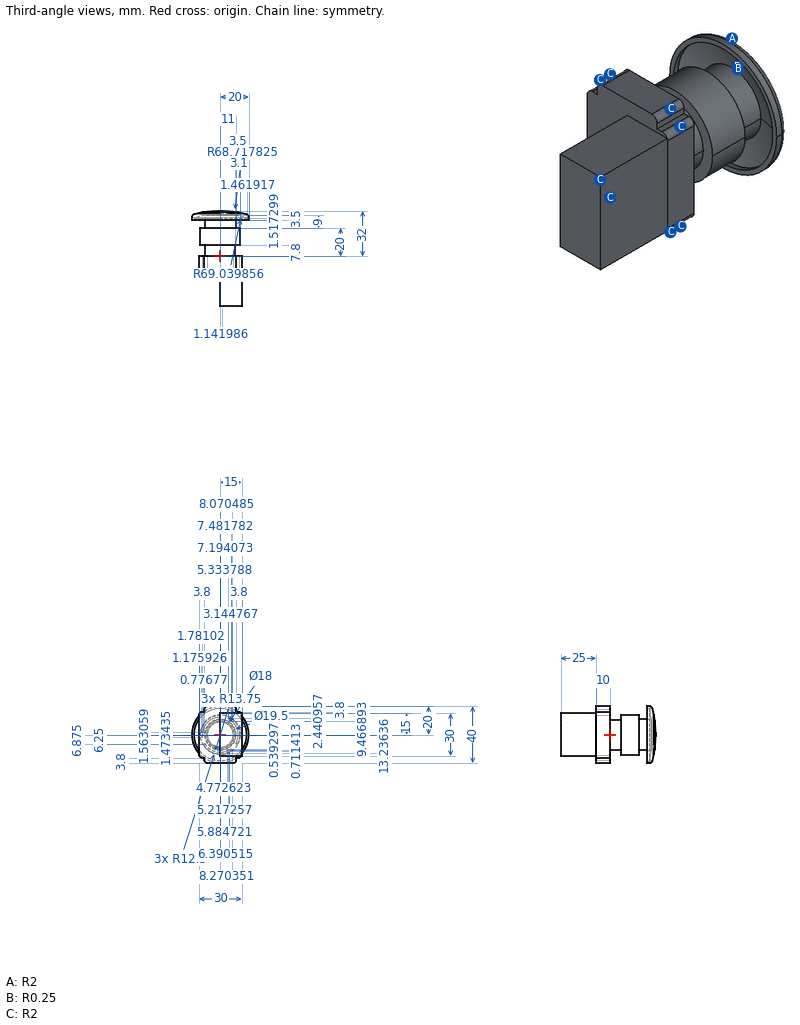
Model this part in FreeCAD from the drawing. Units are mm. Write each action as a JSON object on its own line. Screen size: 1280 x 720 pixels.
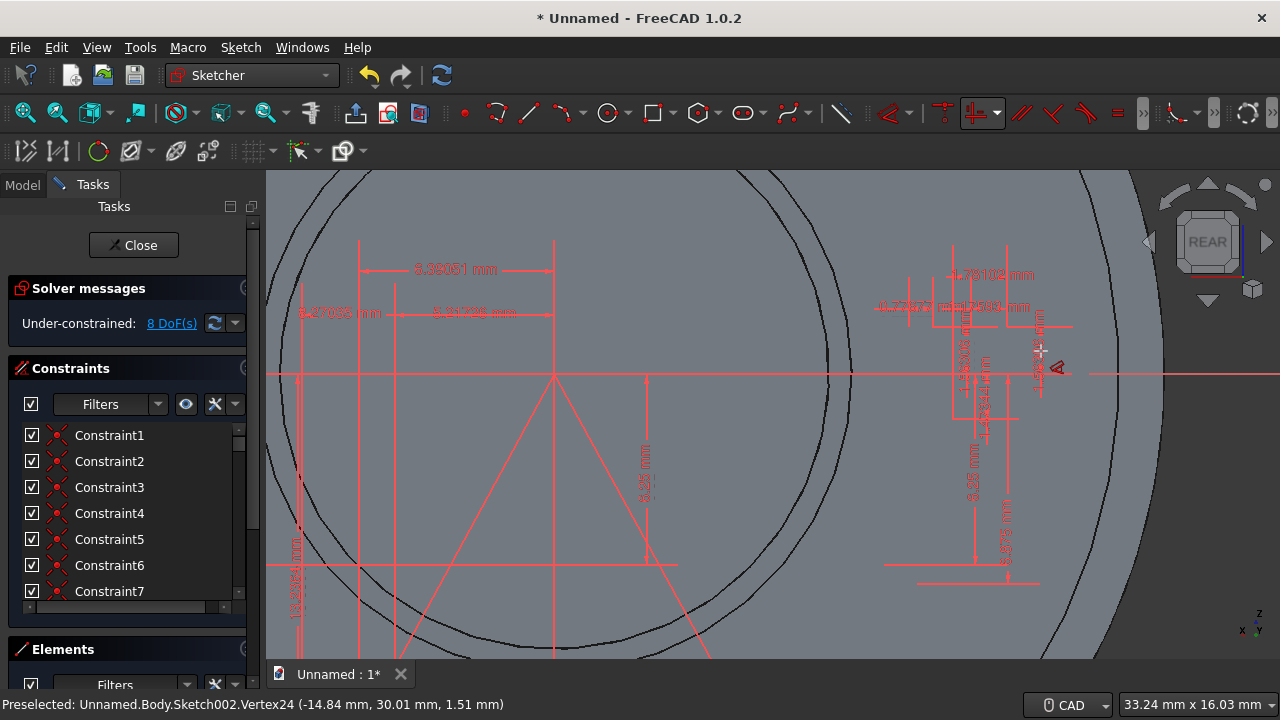
{"action": "scroll", "coordinate": [780, 442], "scroll_direction": "down", "scroll_amount": 5}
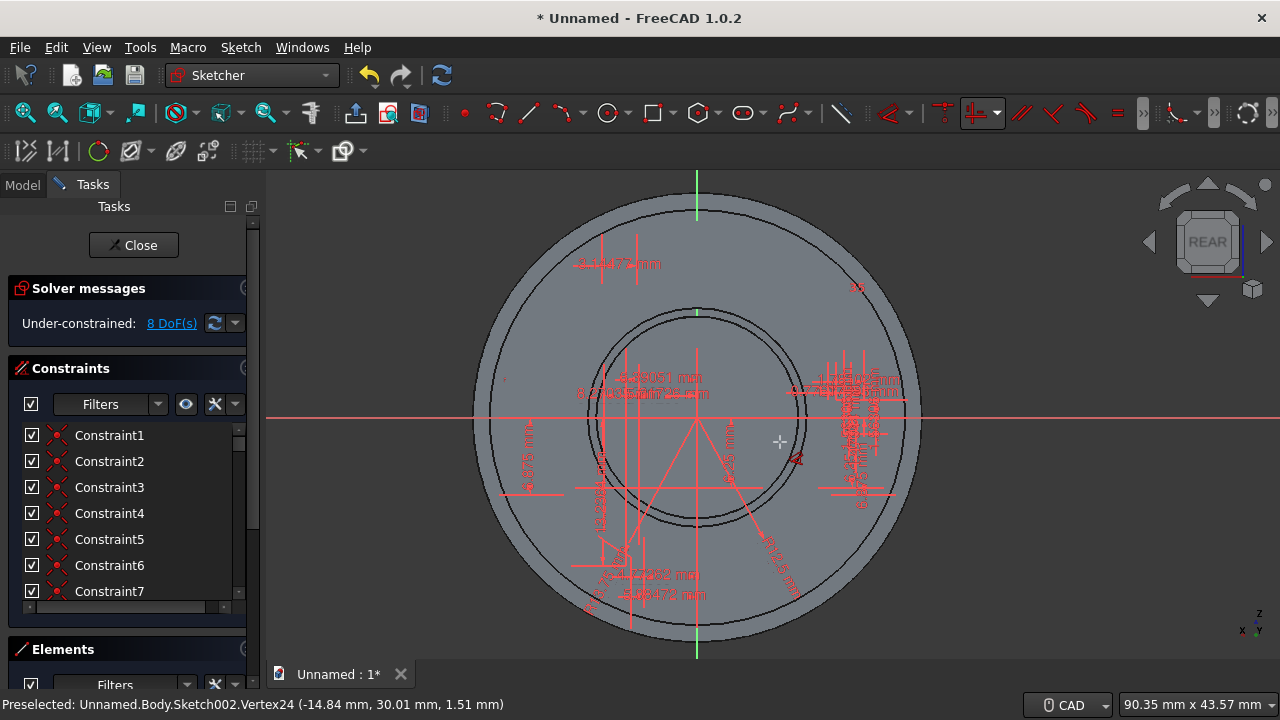
{"action": "scroll", "coordinate": [613, 305], "scroll_direction": "up", "scroll_amount": 3}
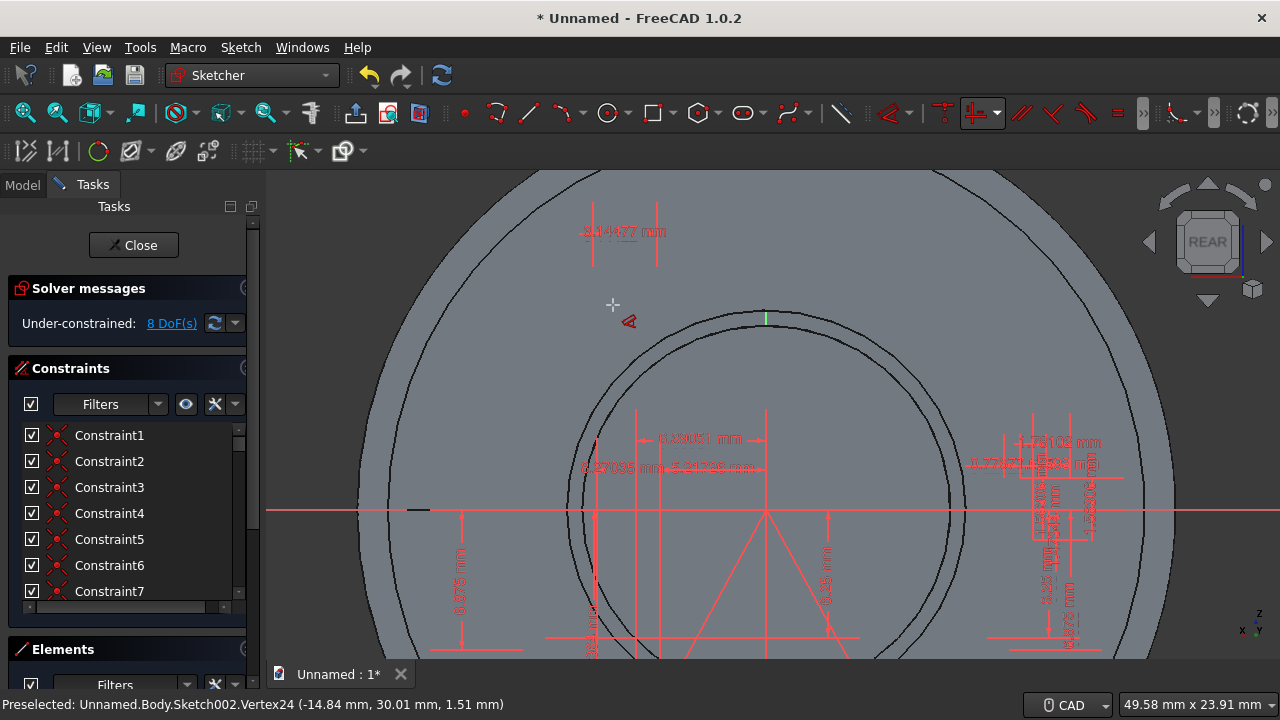
{"action": "left_click", "coordinate": [613, 305]}
{"action": "left_click", "coordinate": [690, 271]}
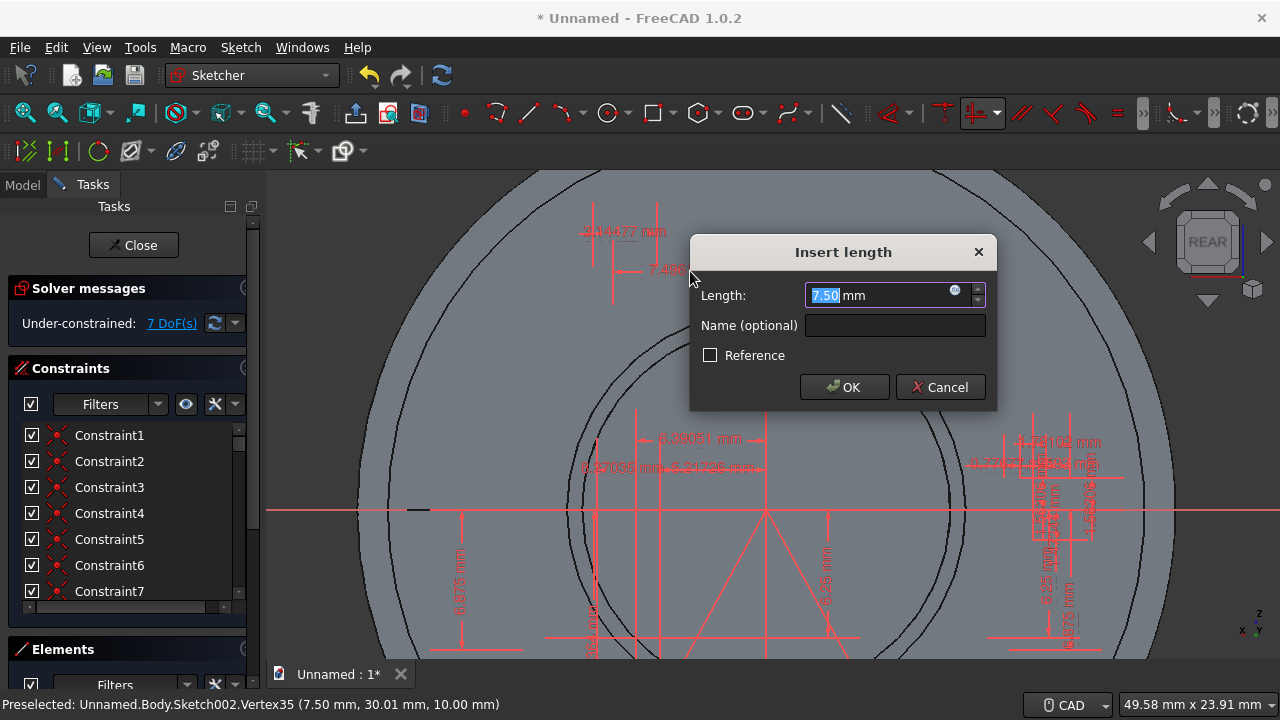
{"action": "type", "text": "7.481782"}
{"action": "key", "text": "Return"}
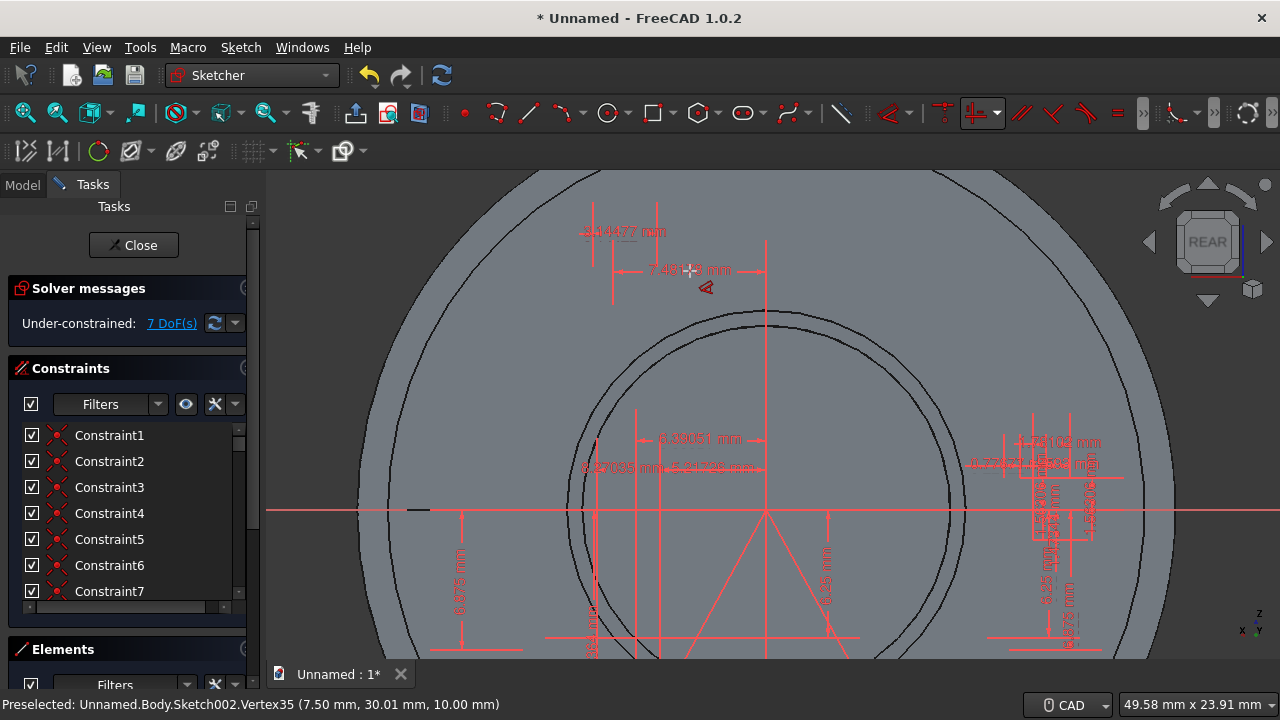
{"action": "left_click", "coordinate": [619, 317]}
{"action": "left_click", "coordinate": [693, 544]}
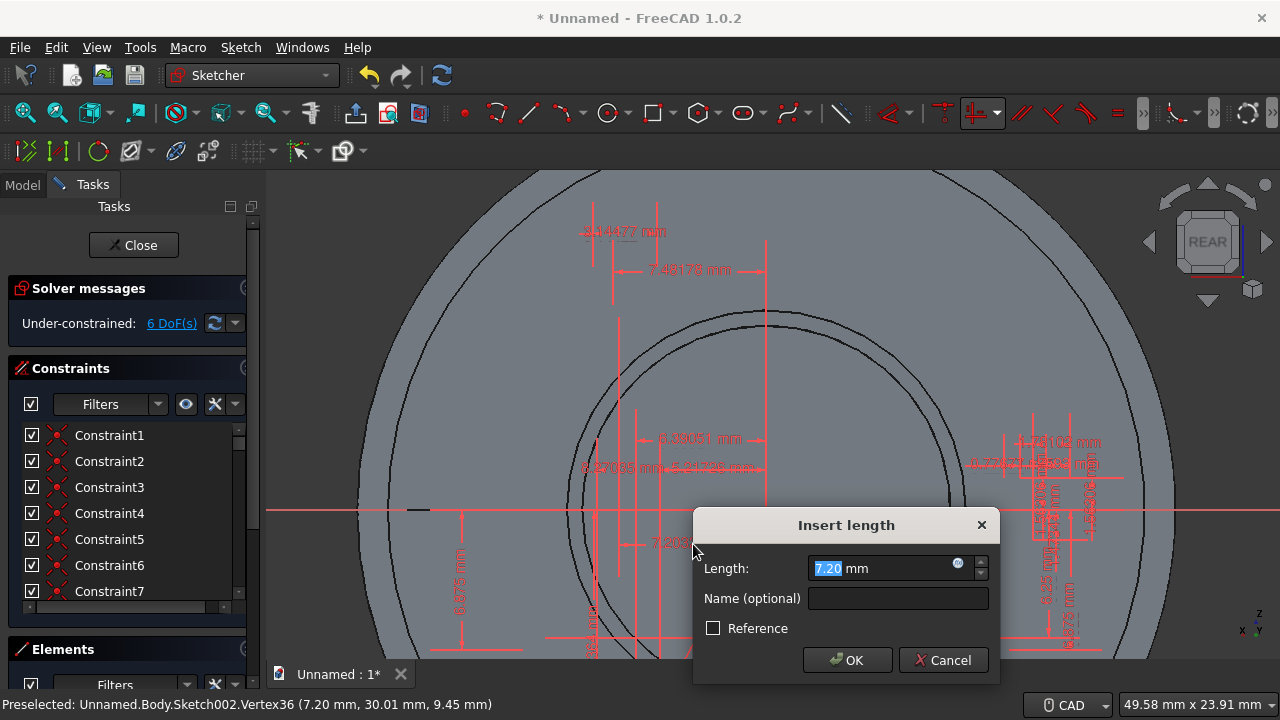
{"action": "type", "text": "7.194073"}
{"action": "key", "text": "Return"}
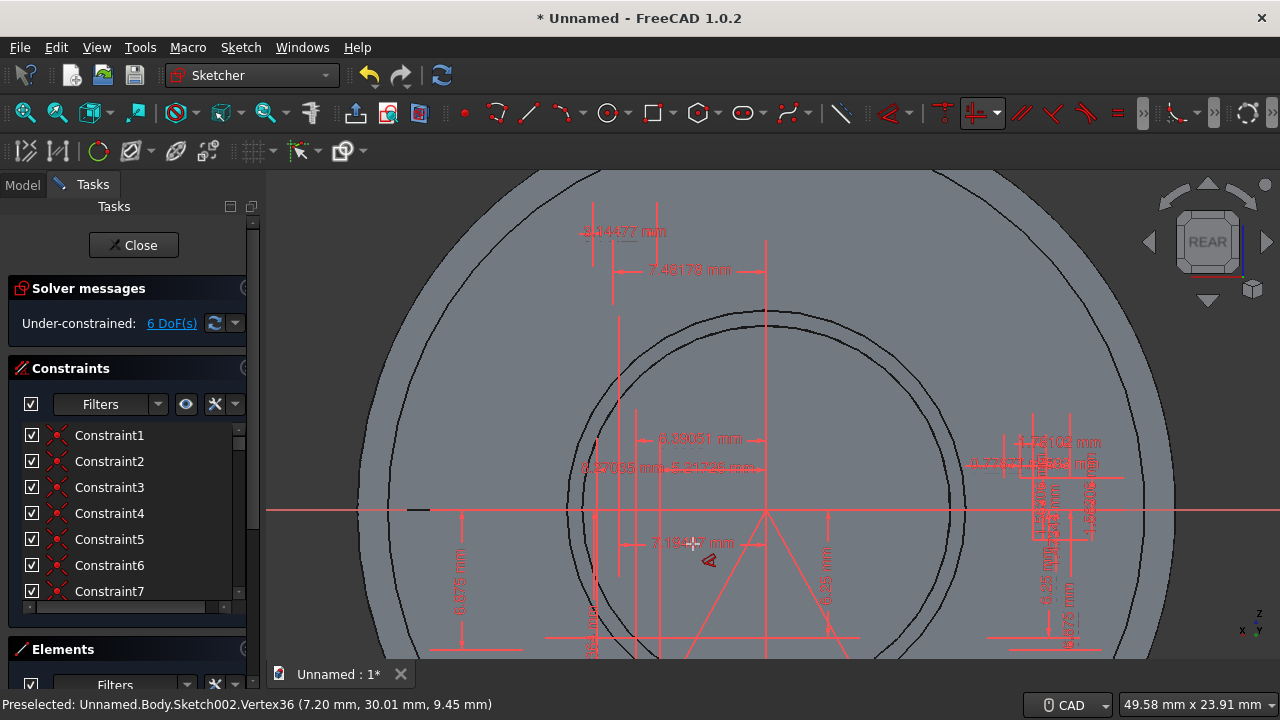
{"action": "left_click", "coordinate": [619, 317]}
{"action": "left_click", "coordinate": [585, 413]}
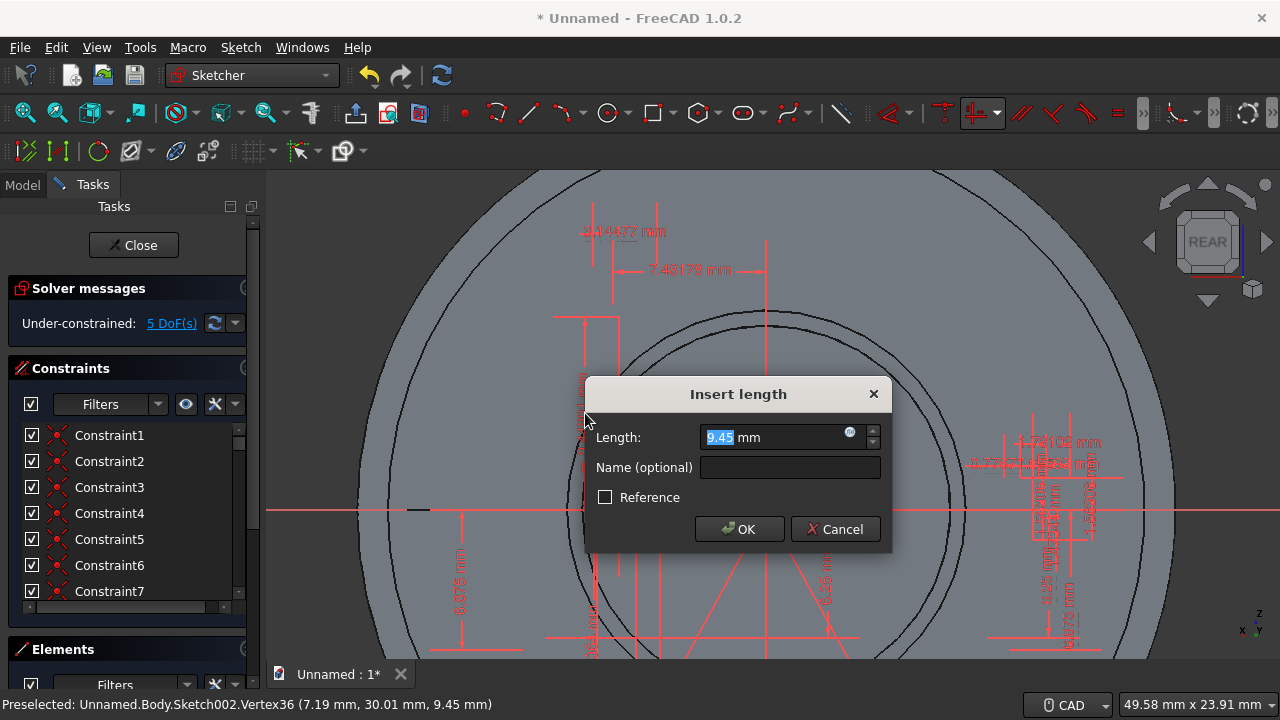
{"action": "type", "text": "9.466893"}
{"action": "key", "text": "Return"}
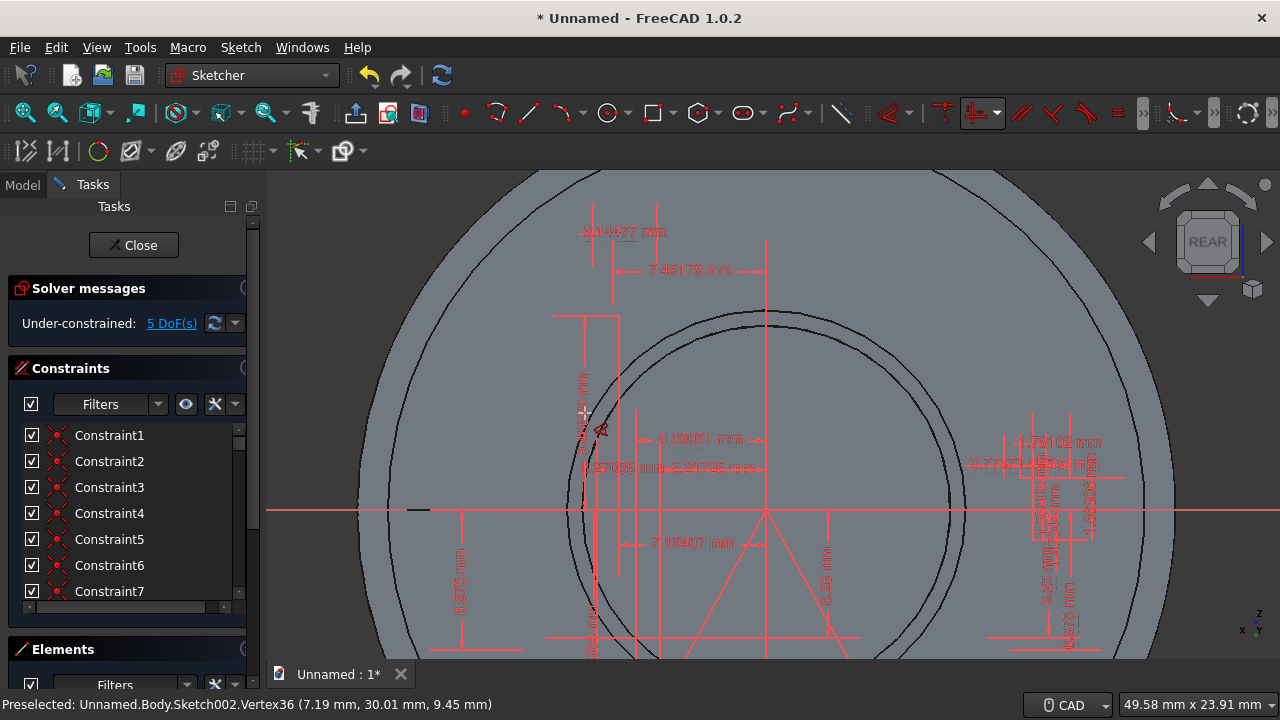
{"action": "left_click", "coordinate": [657, 267]}
{"action": "left_click", "coordinate": [712, 233]}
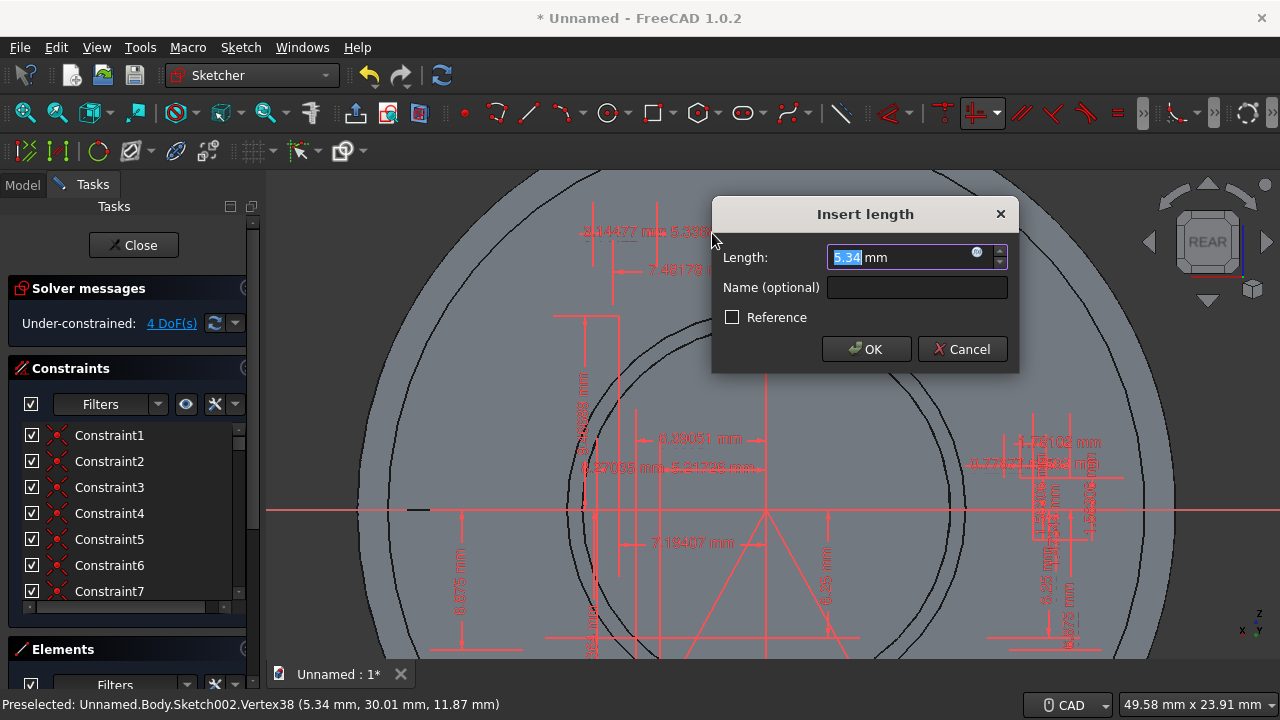
{"action": "type", "text": "5.333788"}
{"action": "key", "text": "Return"}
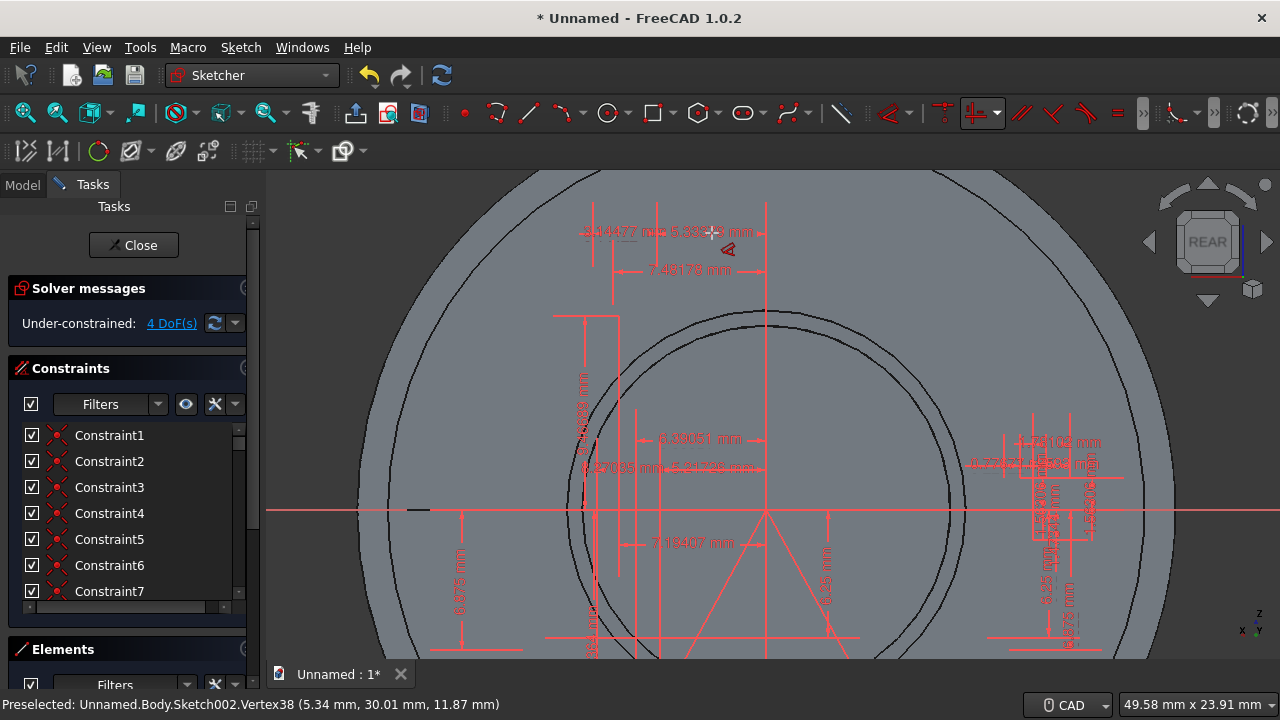
{"action": "left_click", "coordinate": [602, 282]}
{"action": "left_click", "coordinate": [684, 568]}